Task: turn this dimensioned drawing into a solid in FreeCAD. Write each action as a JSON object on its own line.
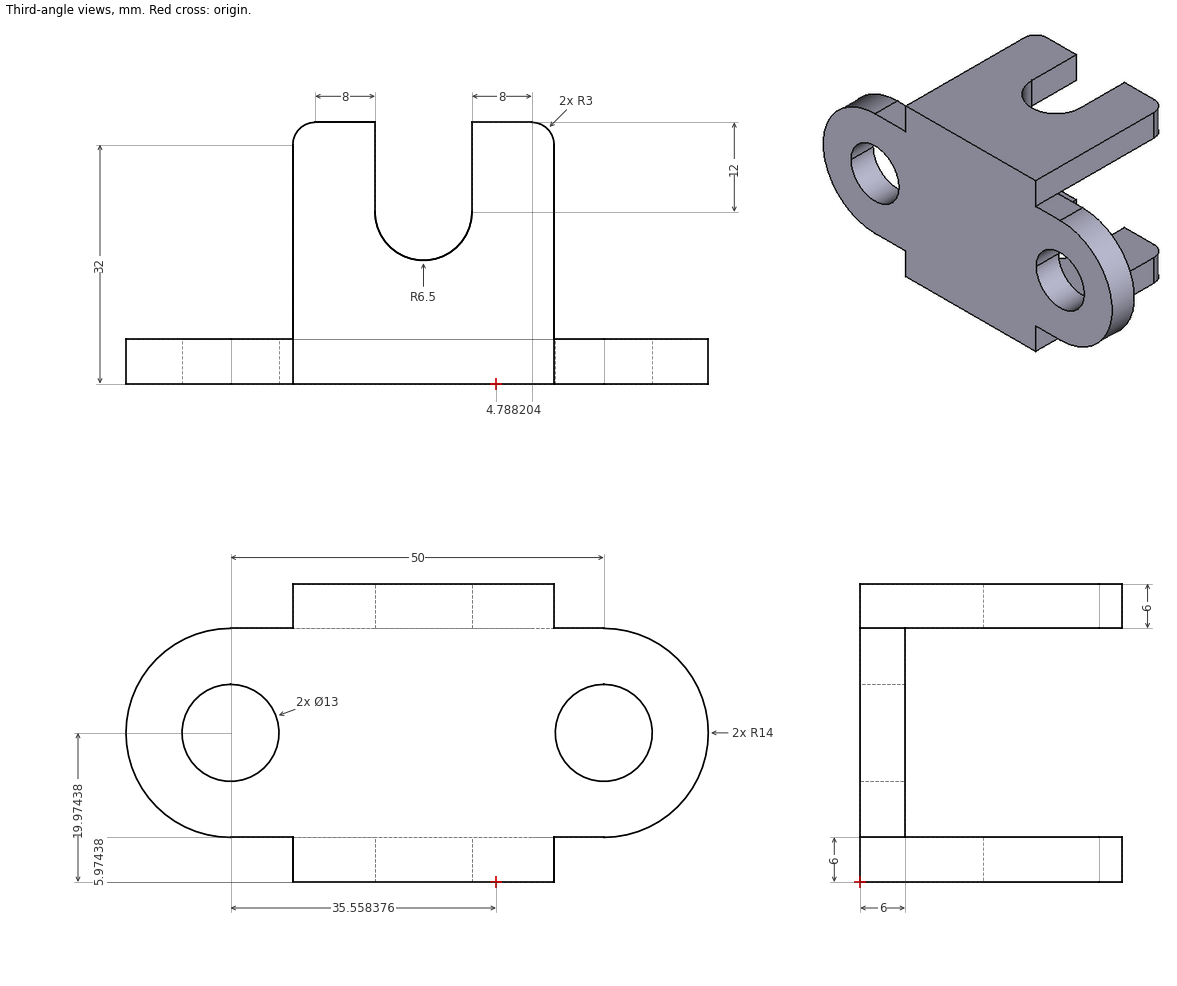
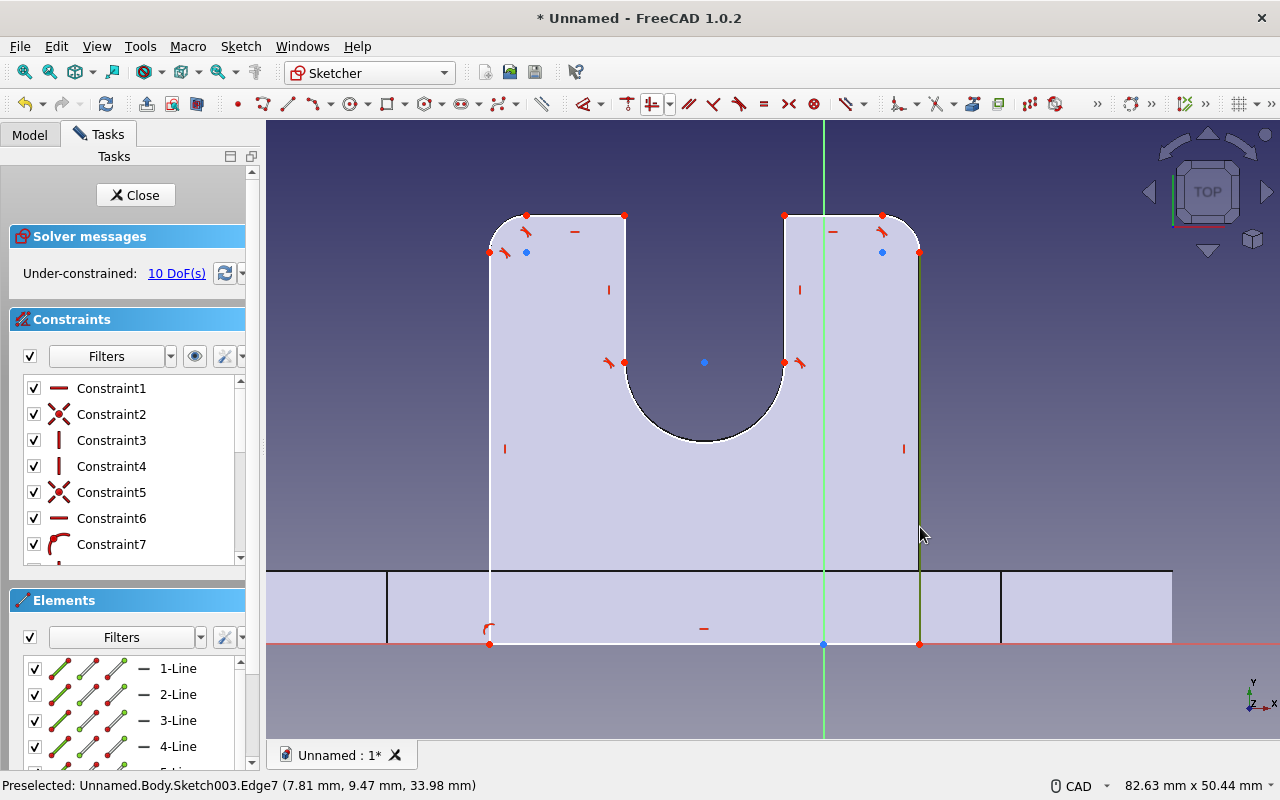
{"action": "left_click", "coordinate": [916, 236]}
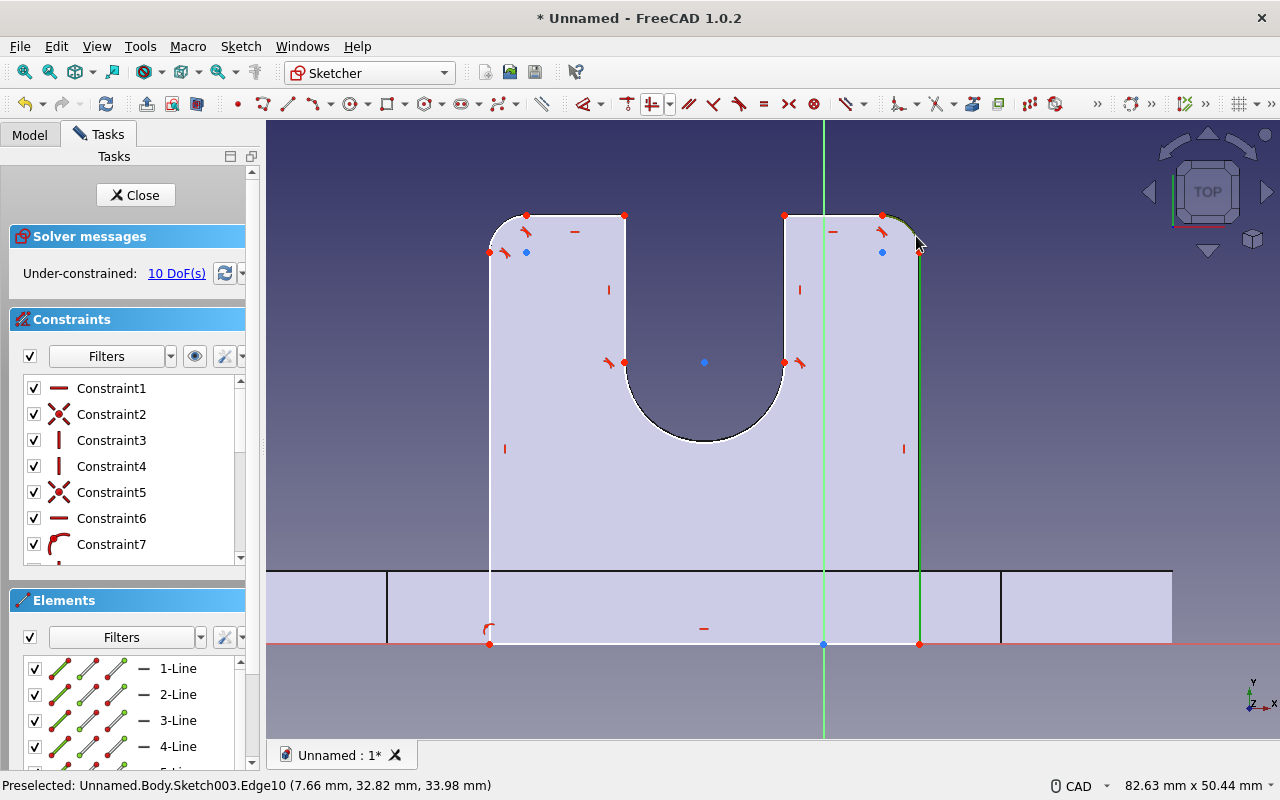
{"action": "left_click", "coordinate": [739, 104]}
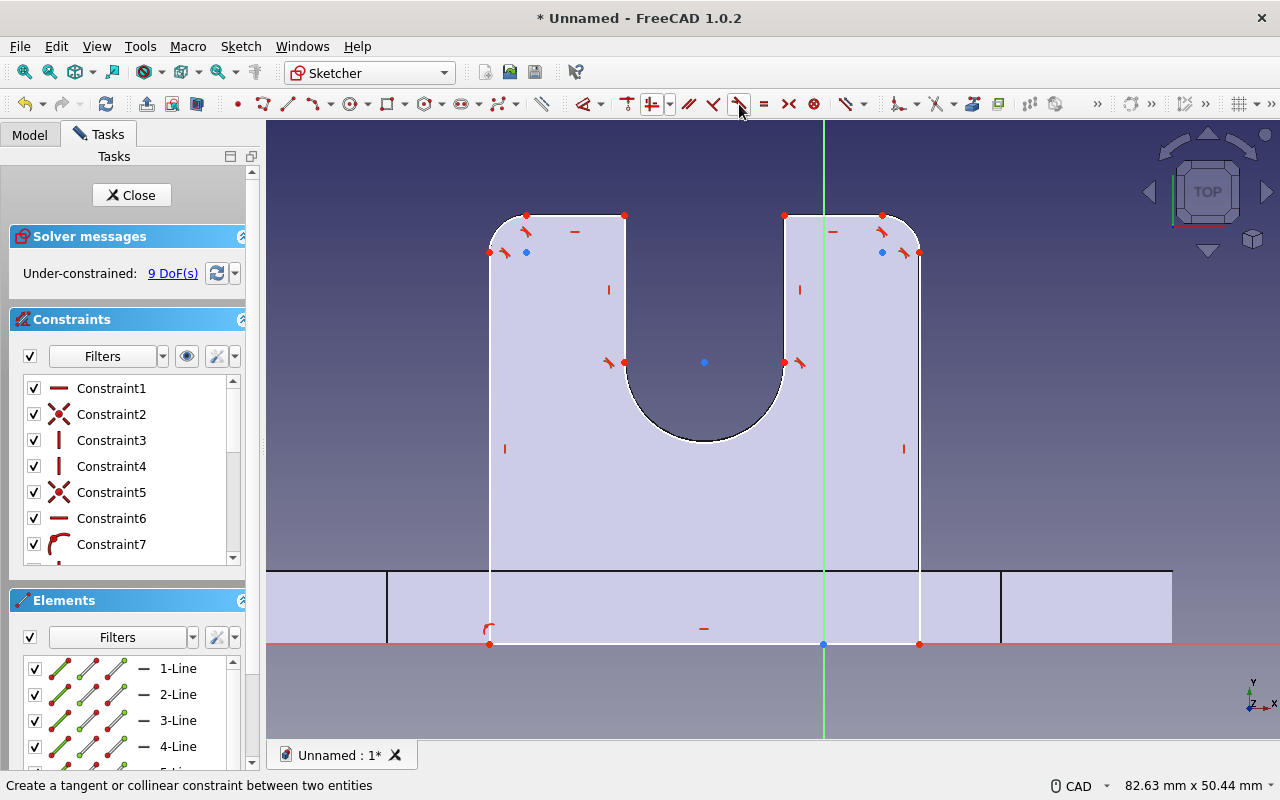
{"action": "left_click", "coordinate": [510, 220]}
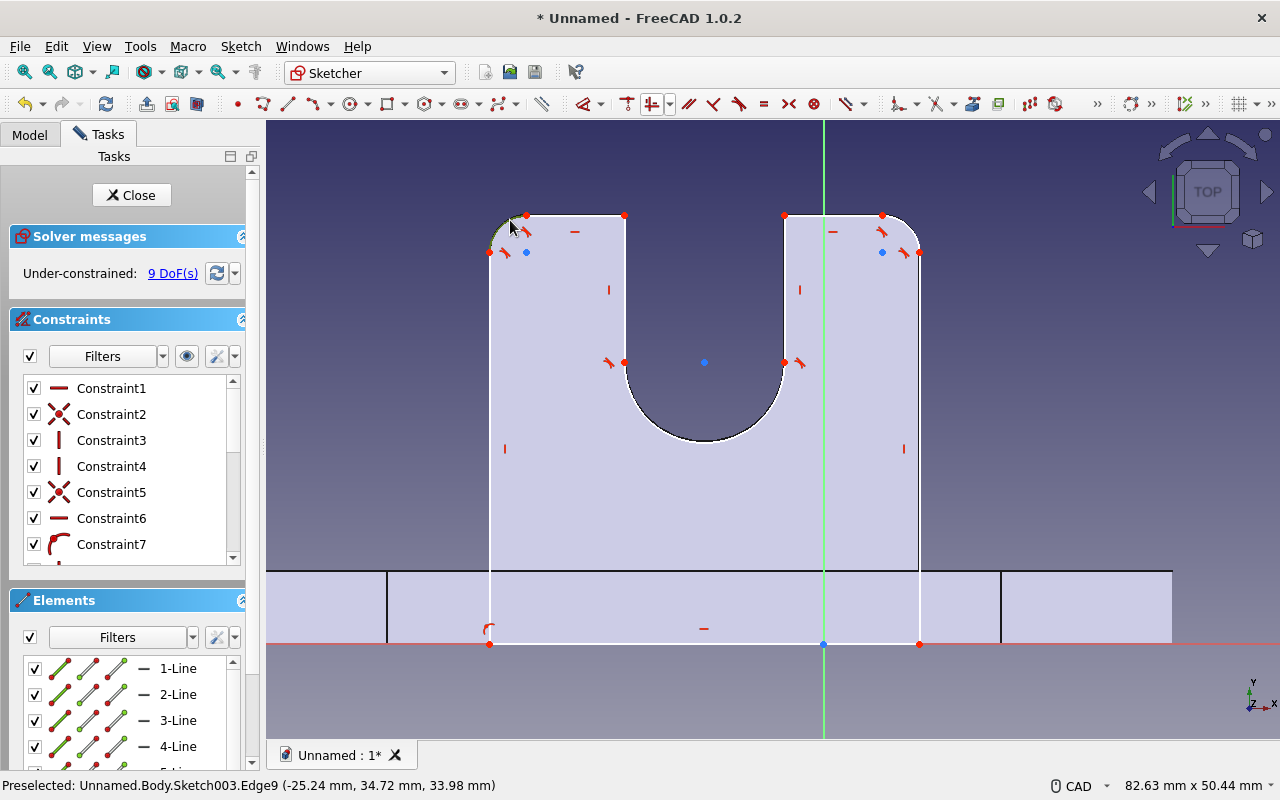
{"action": "left_click", "coordinate": [916, 236]}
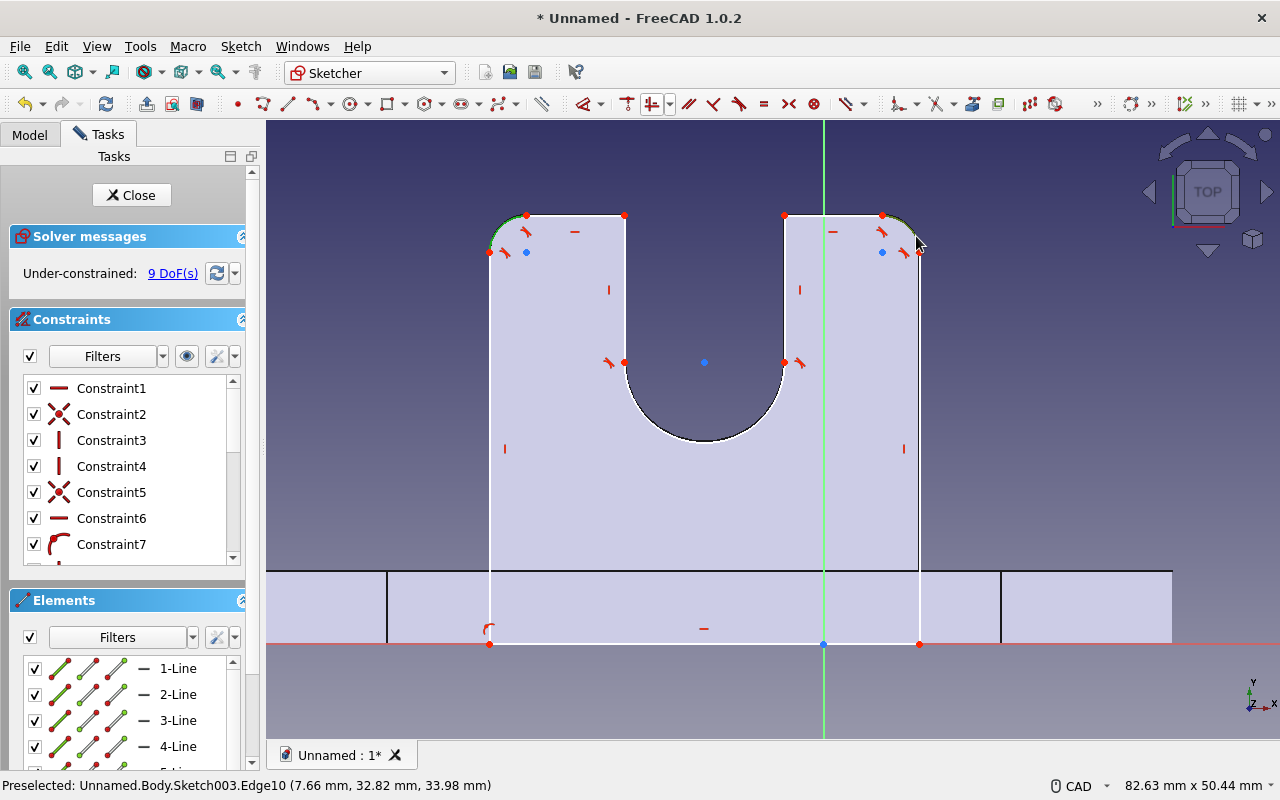
{"action": "left_click", "coordinate": [764, 104]}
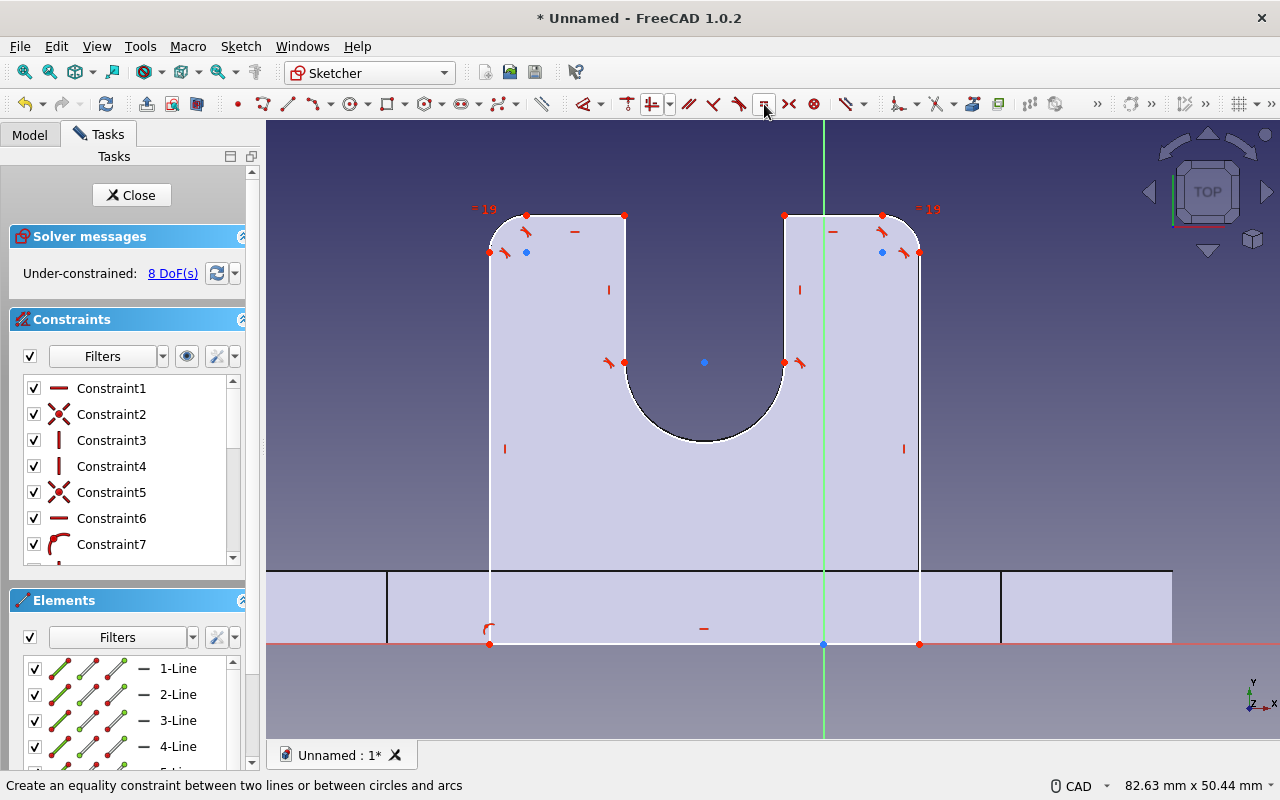
{"action": "left_click", "coordinate": [582, 104]}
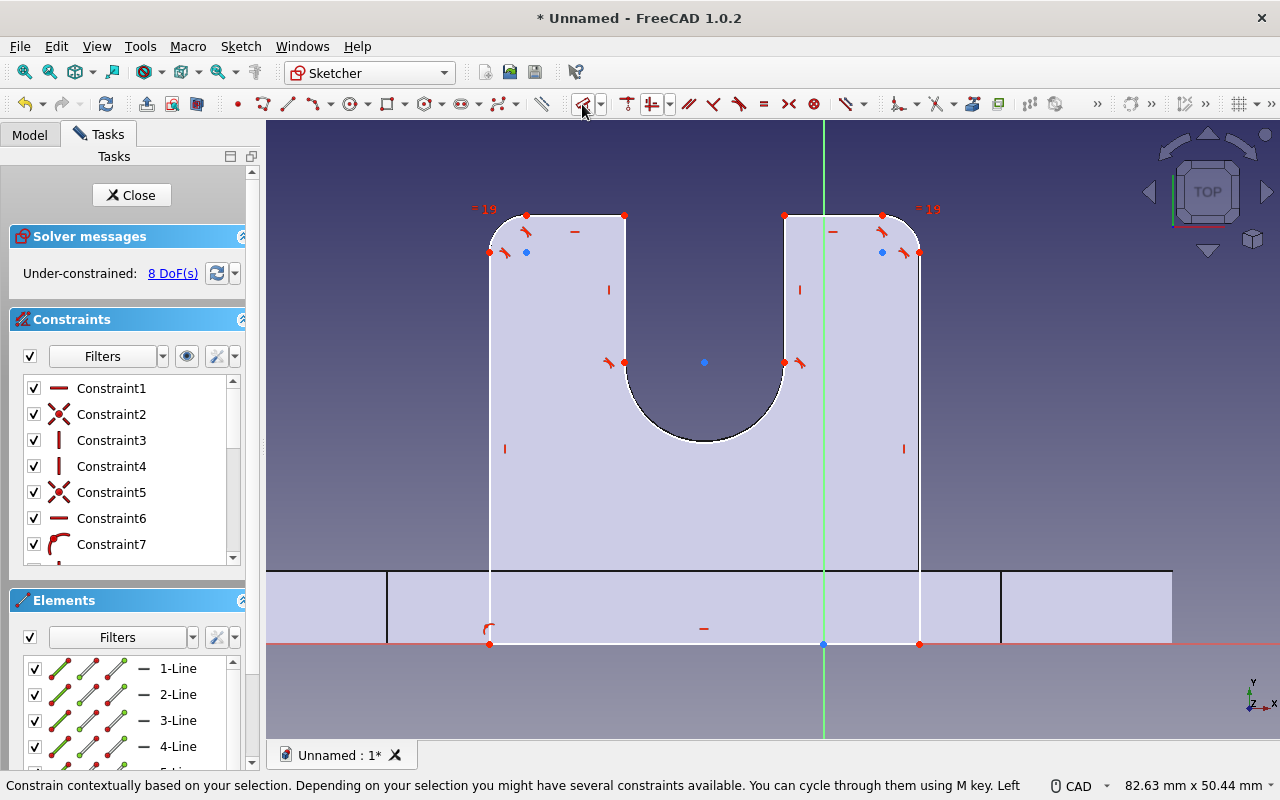
{"action": "left_click", "coordinate": [658, 428]}
{"action": "left_click", "coordinate": [639, 454]}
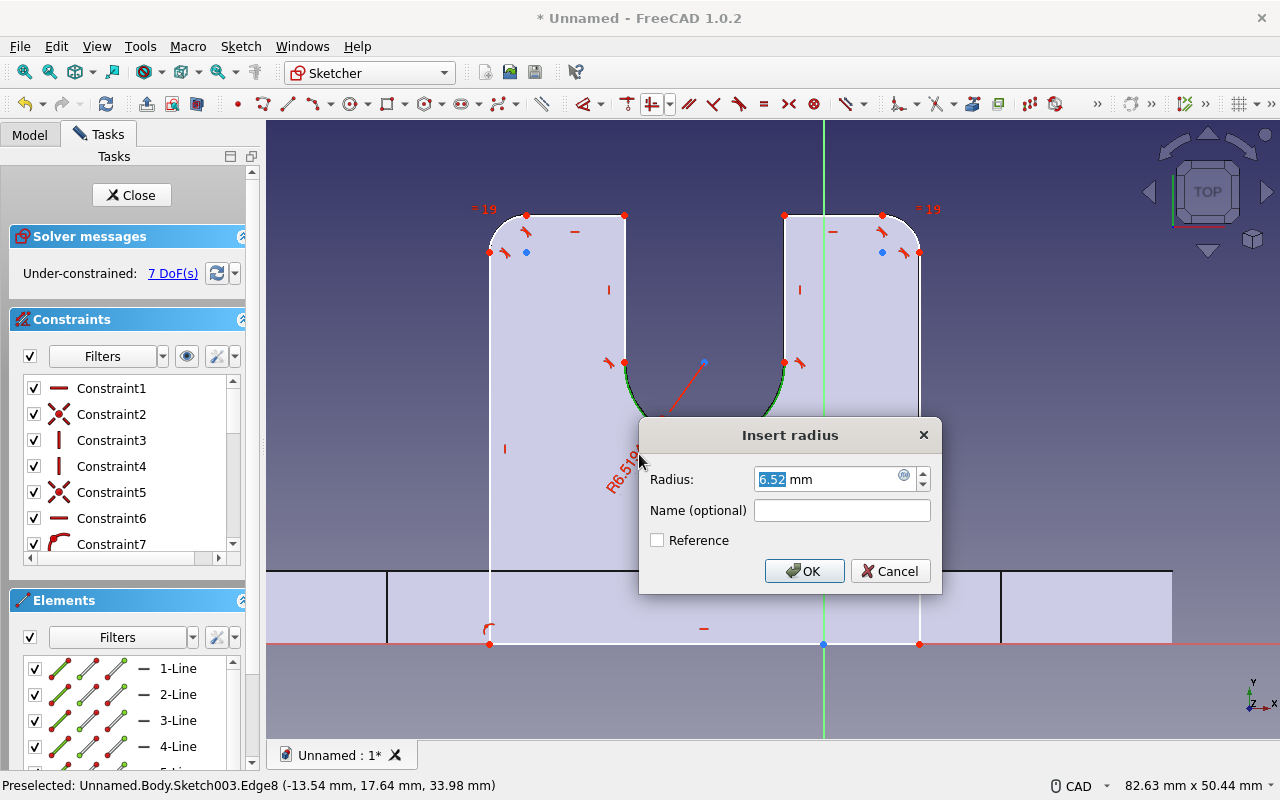
{"action": "type", "text": "6.5"}
{"action": "key", "text": "Return"}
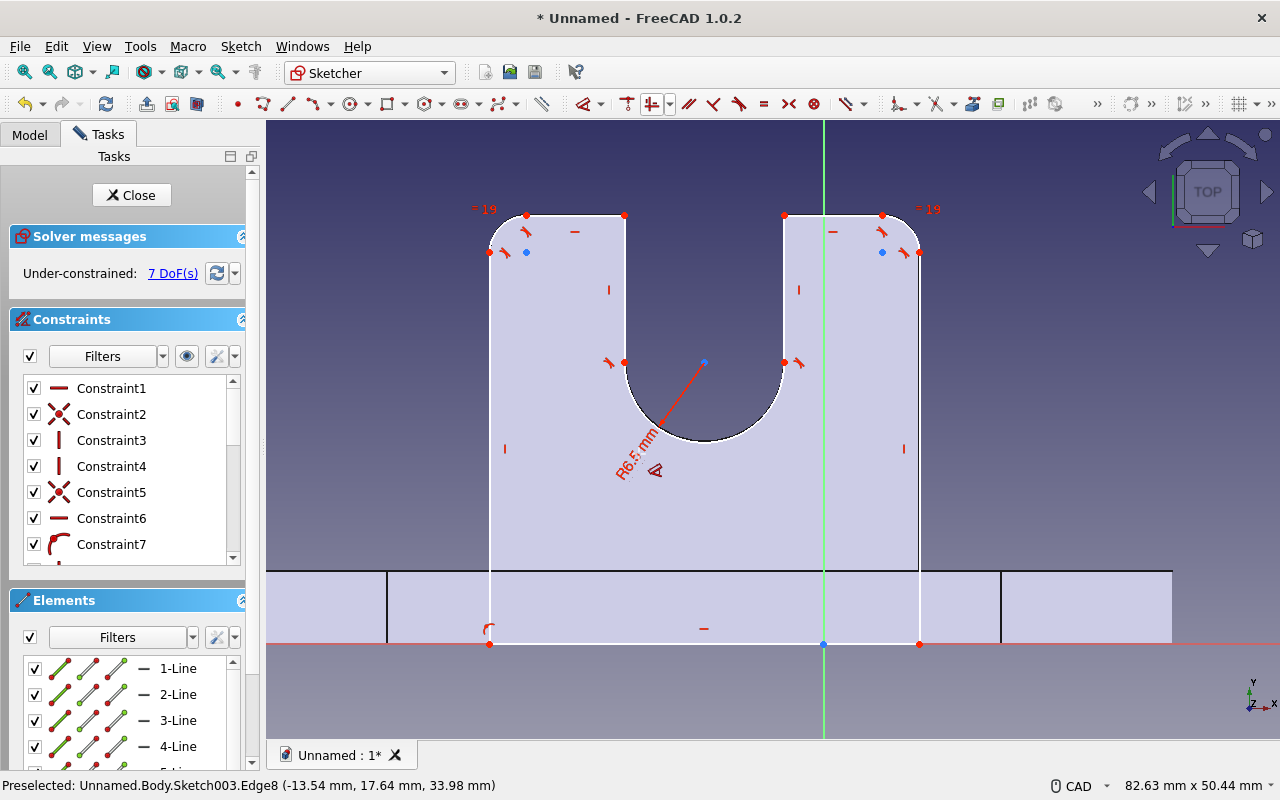
{"action": "left_click", "coordinate": [510, 220]}
{"action": "left_click", "coordinate": [496, 191]}